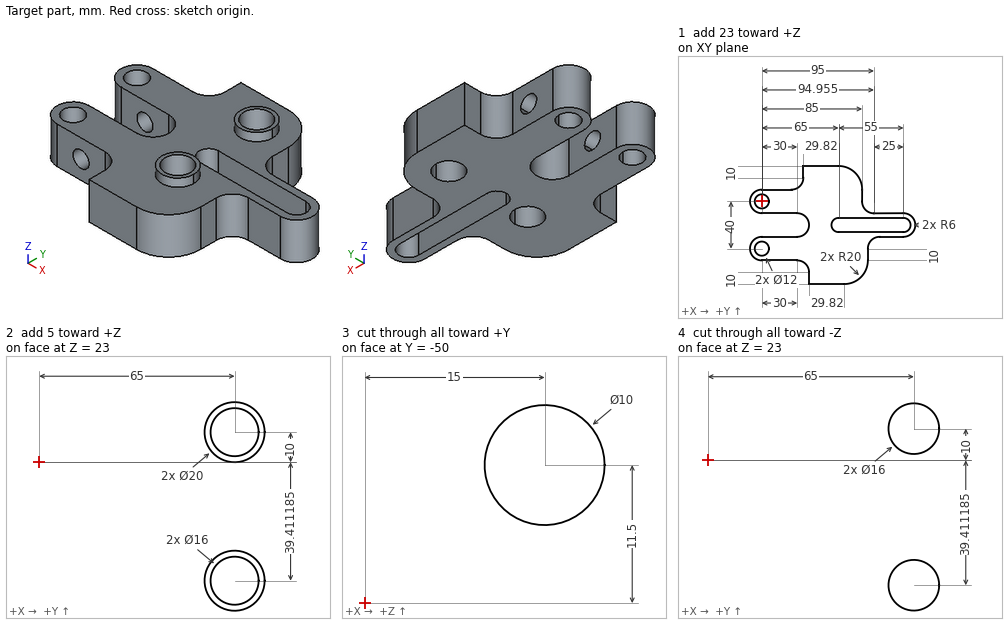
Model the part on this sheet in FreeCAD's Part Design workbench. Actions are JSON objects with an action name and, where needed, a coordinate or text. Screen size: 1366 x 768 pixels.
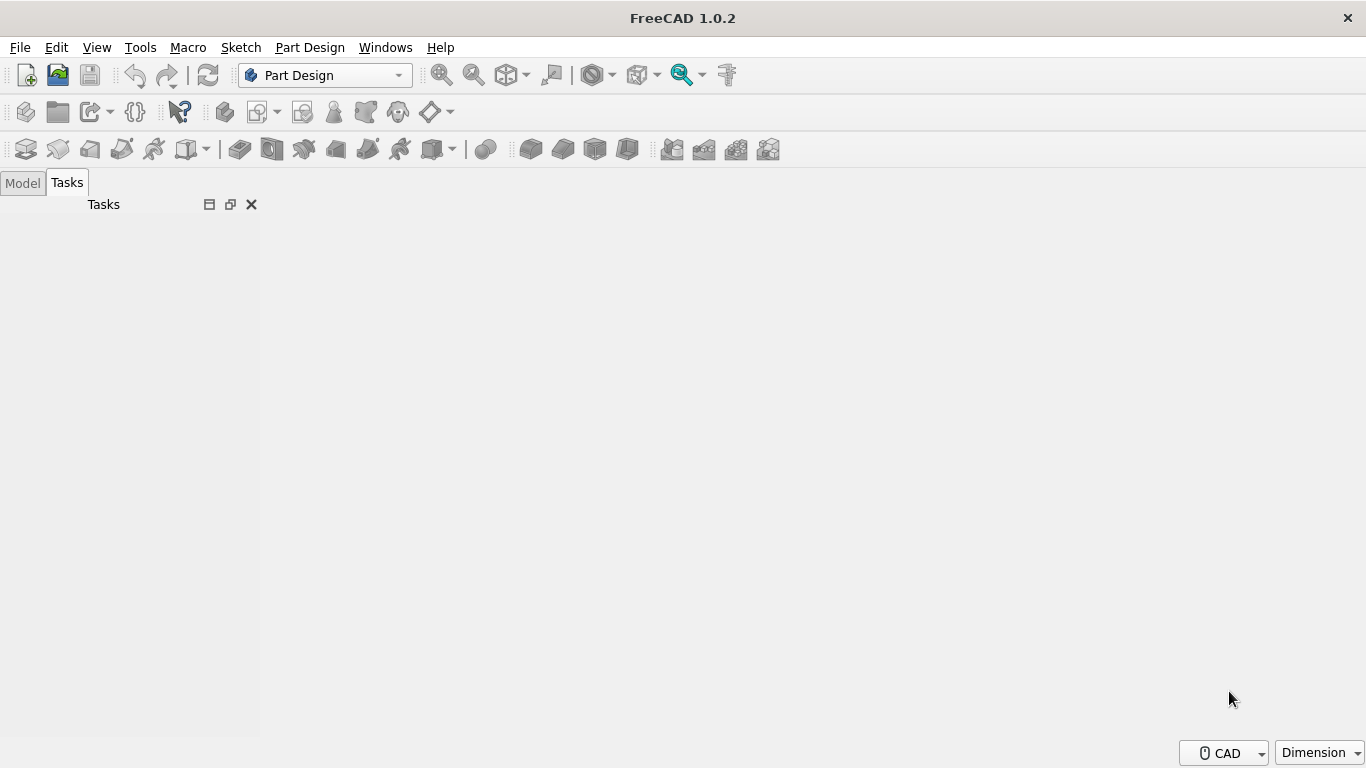
{"action": "left_click", "coordinate": [26, 76]}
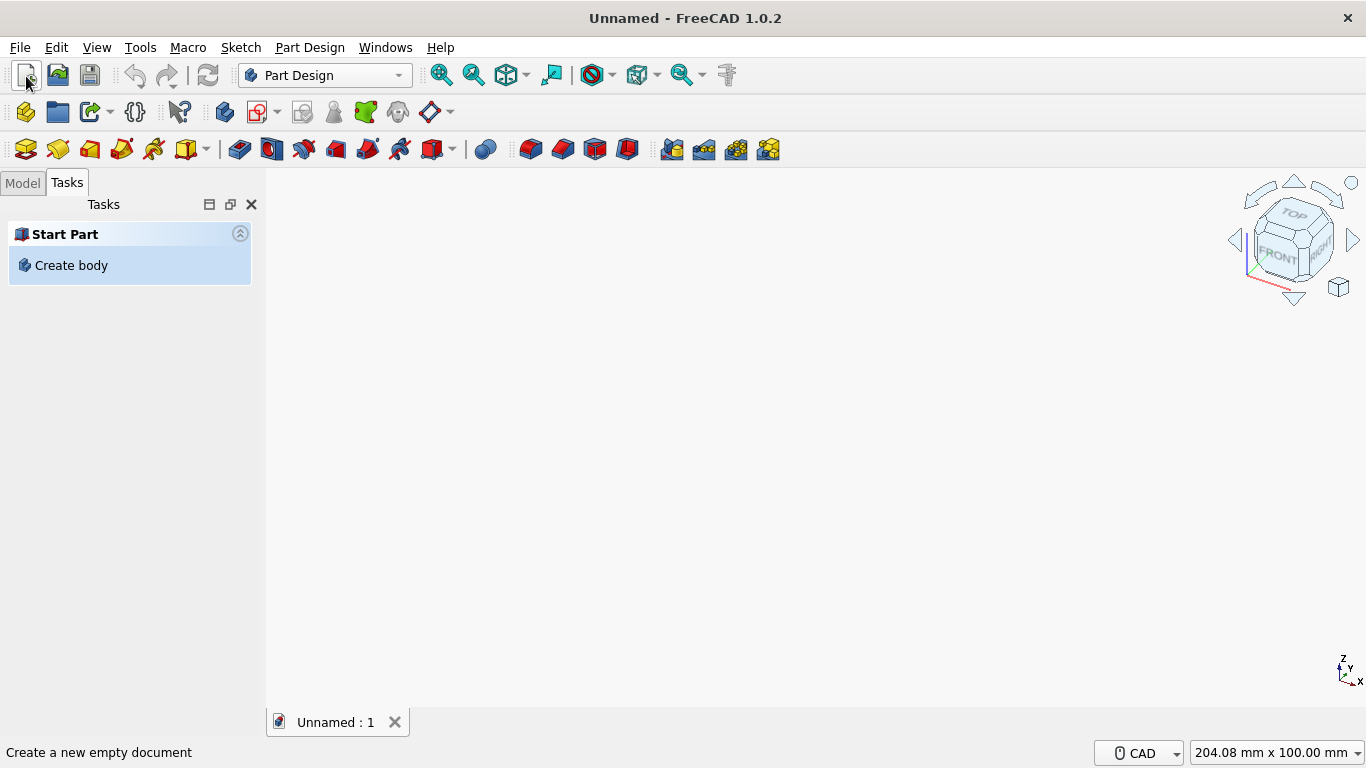
{"action": "left_click", "coordinate": [258, 112]}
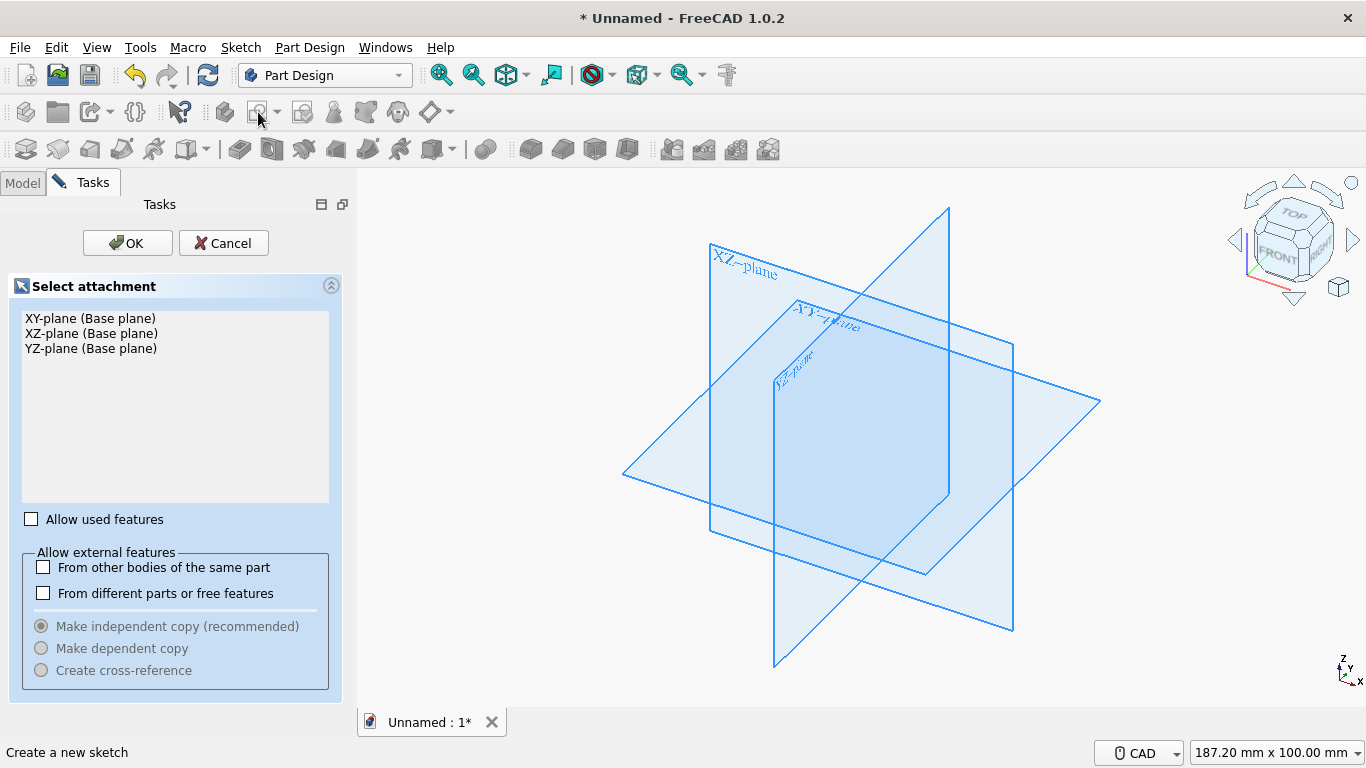
{"action": "left_click", "coordinate": [82, 318]}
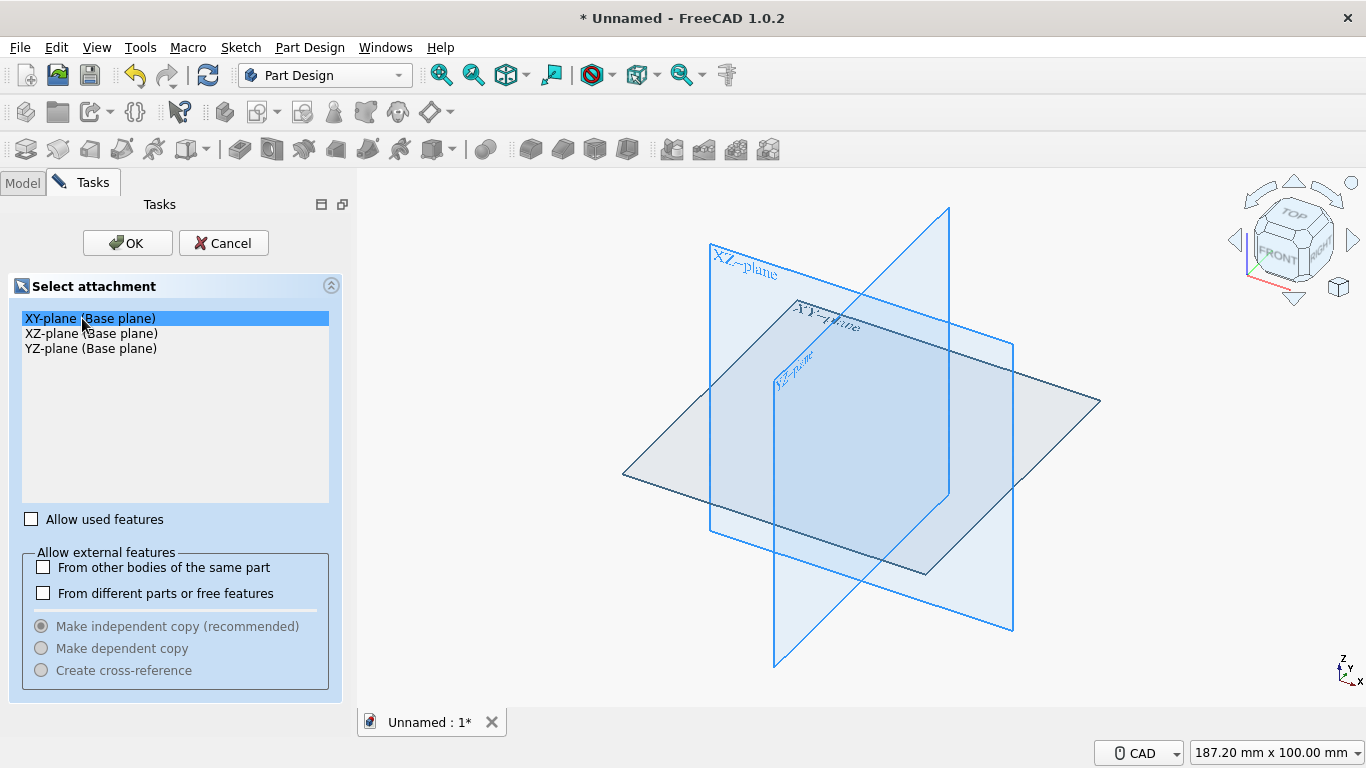
{"action": "left_click", "coordinate": [128, 243]}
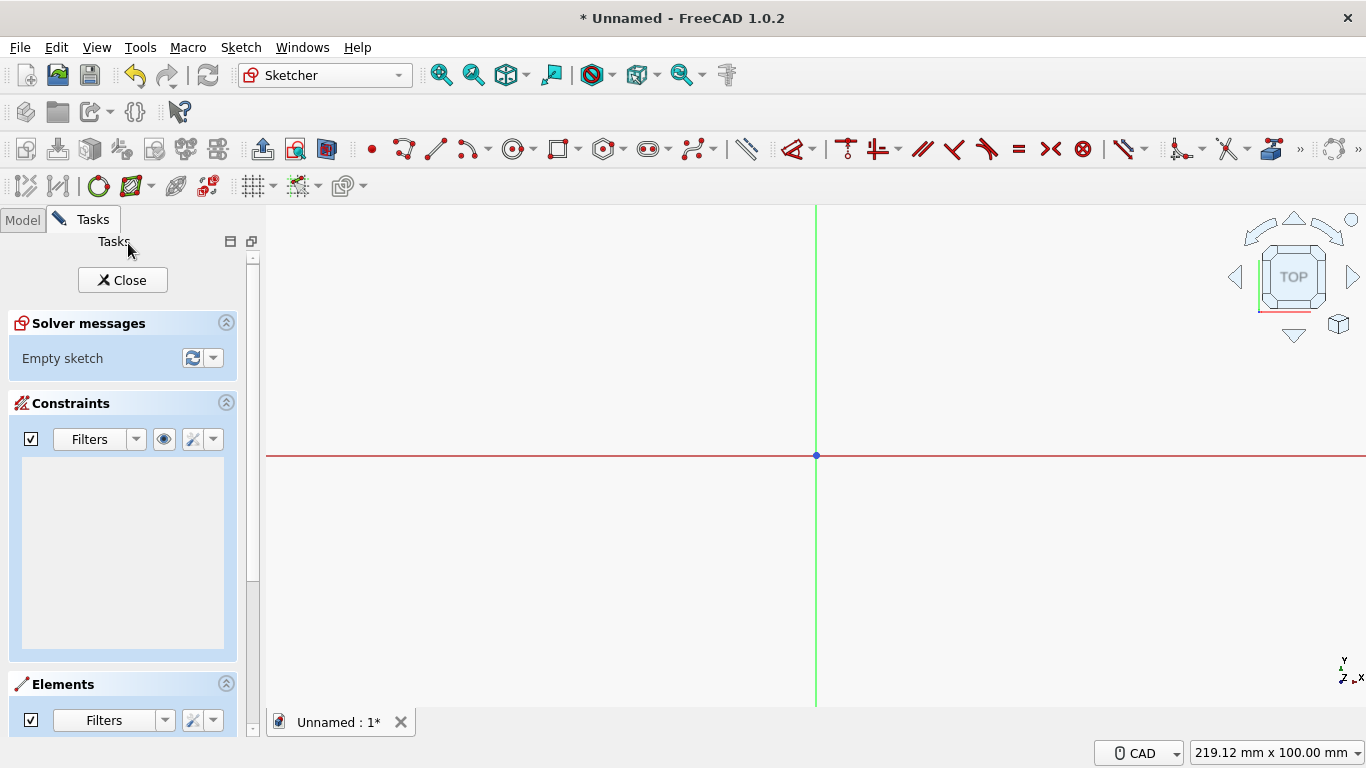
{"action": "scroll", "coordinate": [294, 252], "scroll_direction": "down", "scroll_amount": 2}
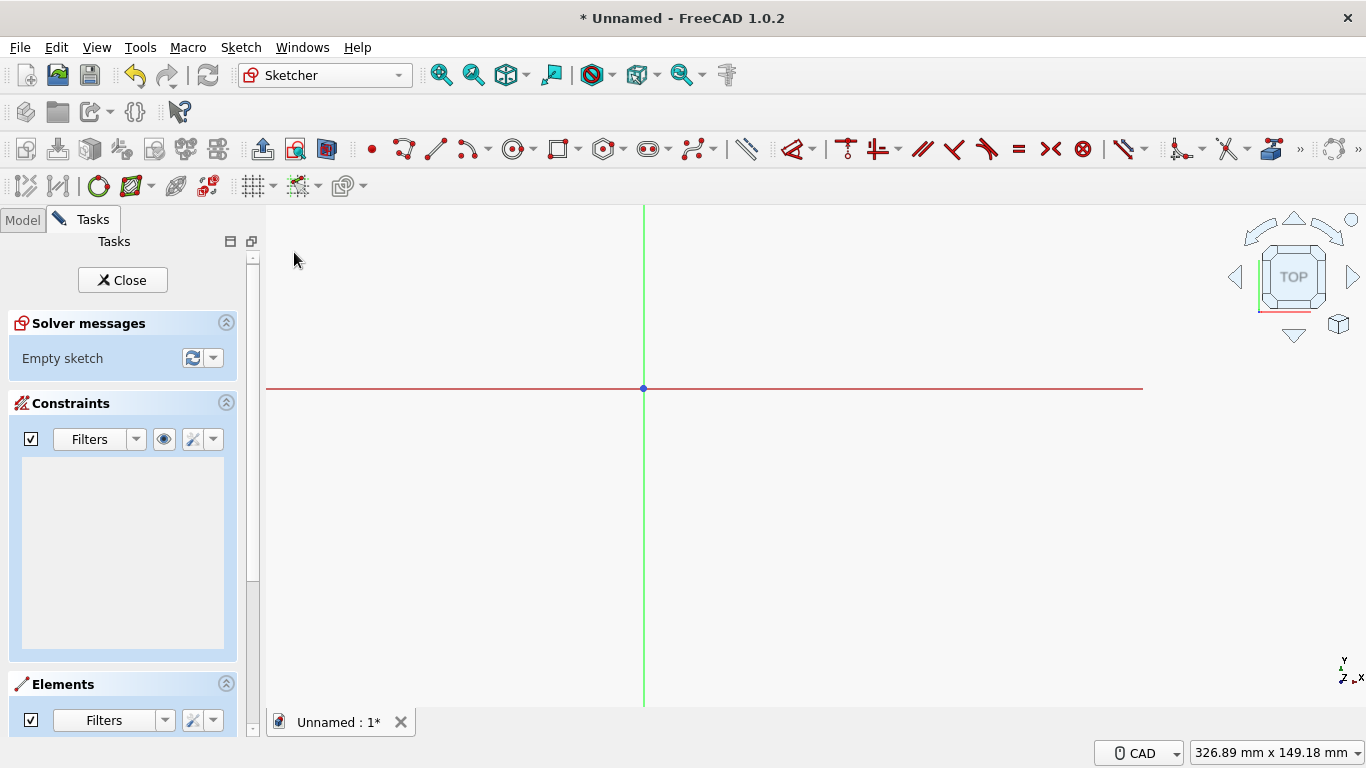
{"action": "left_click", "coordinate": [404, 150]}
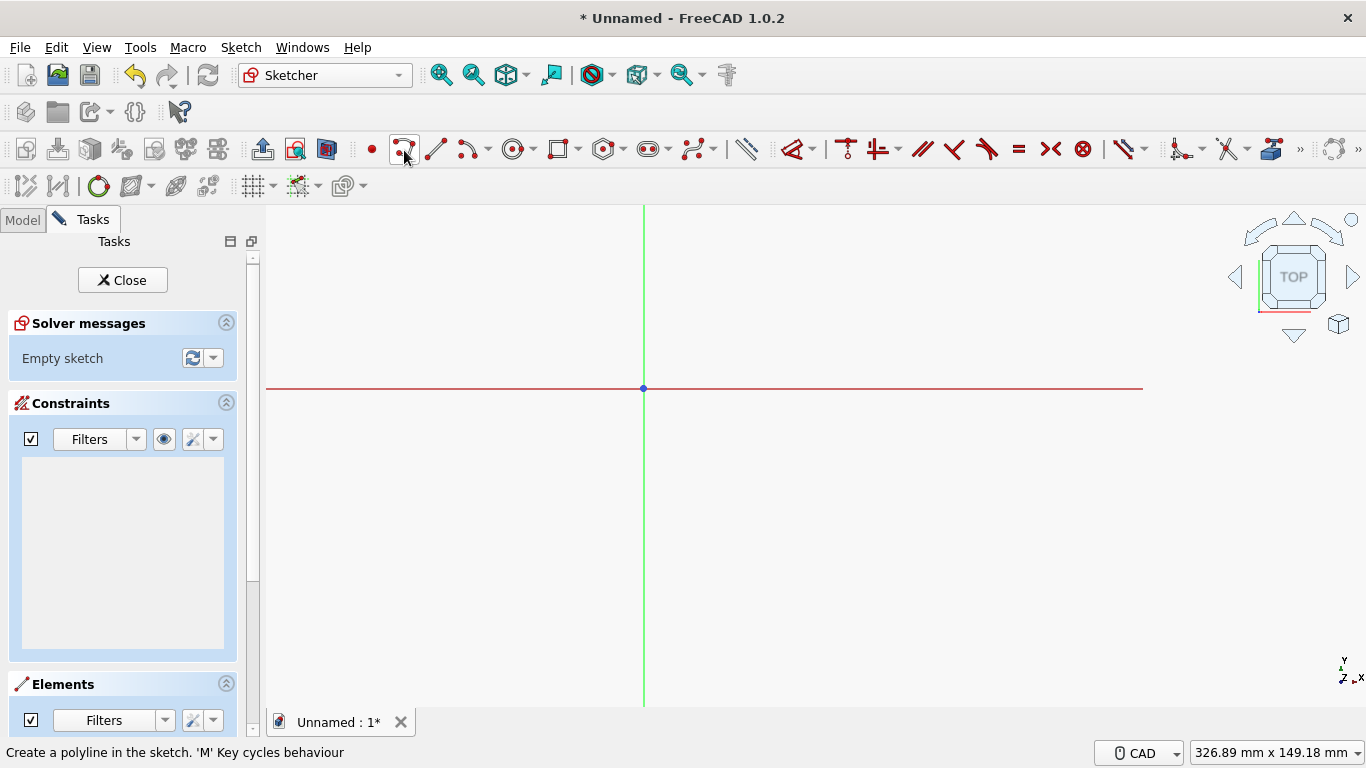
{"action": "left_click", "coordinate": [779, 591]}
{"action": "left_click", "coordinate": [779, 624]}
{"action": "left_click", "coordinate": [879, 624]}
{"action": "right_click", "coordinate": [879, 624]}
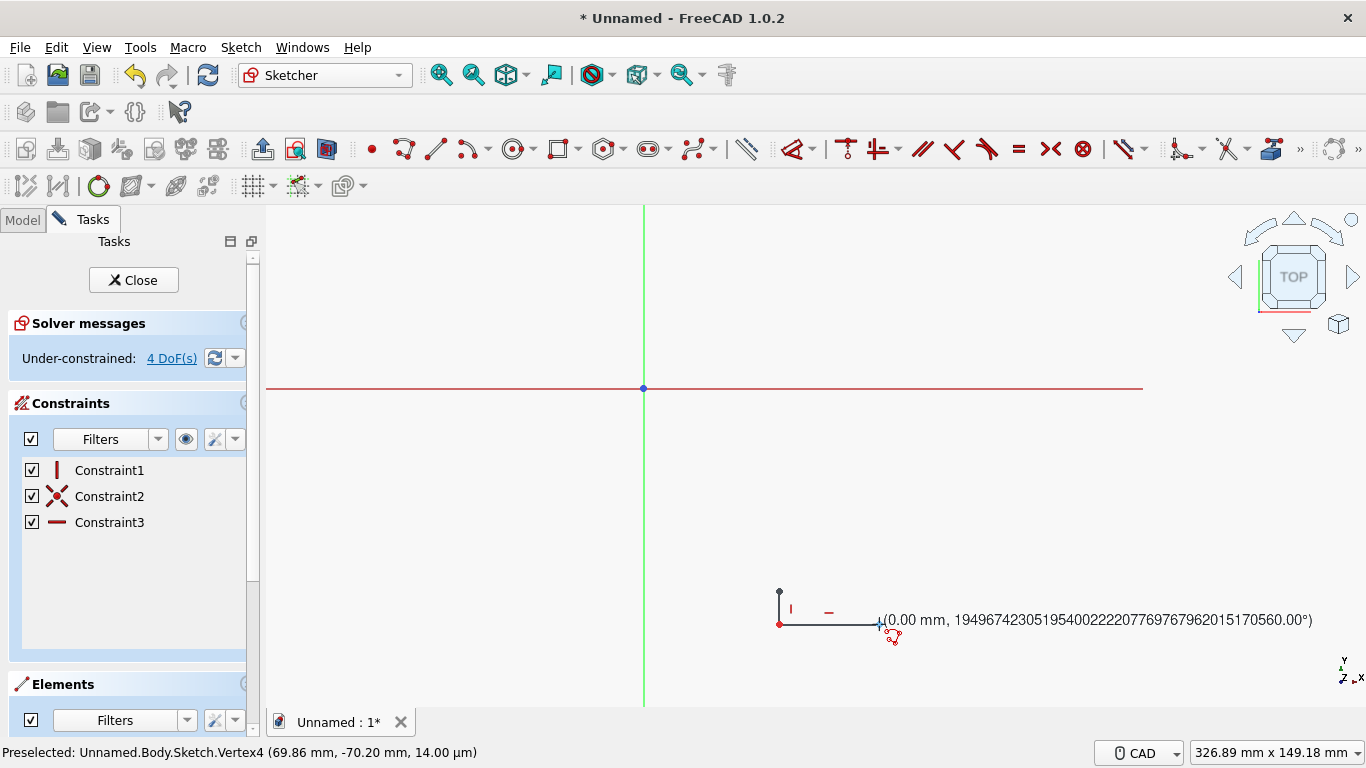
{"action": "key", "text": "g l"}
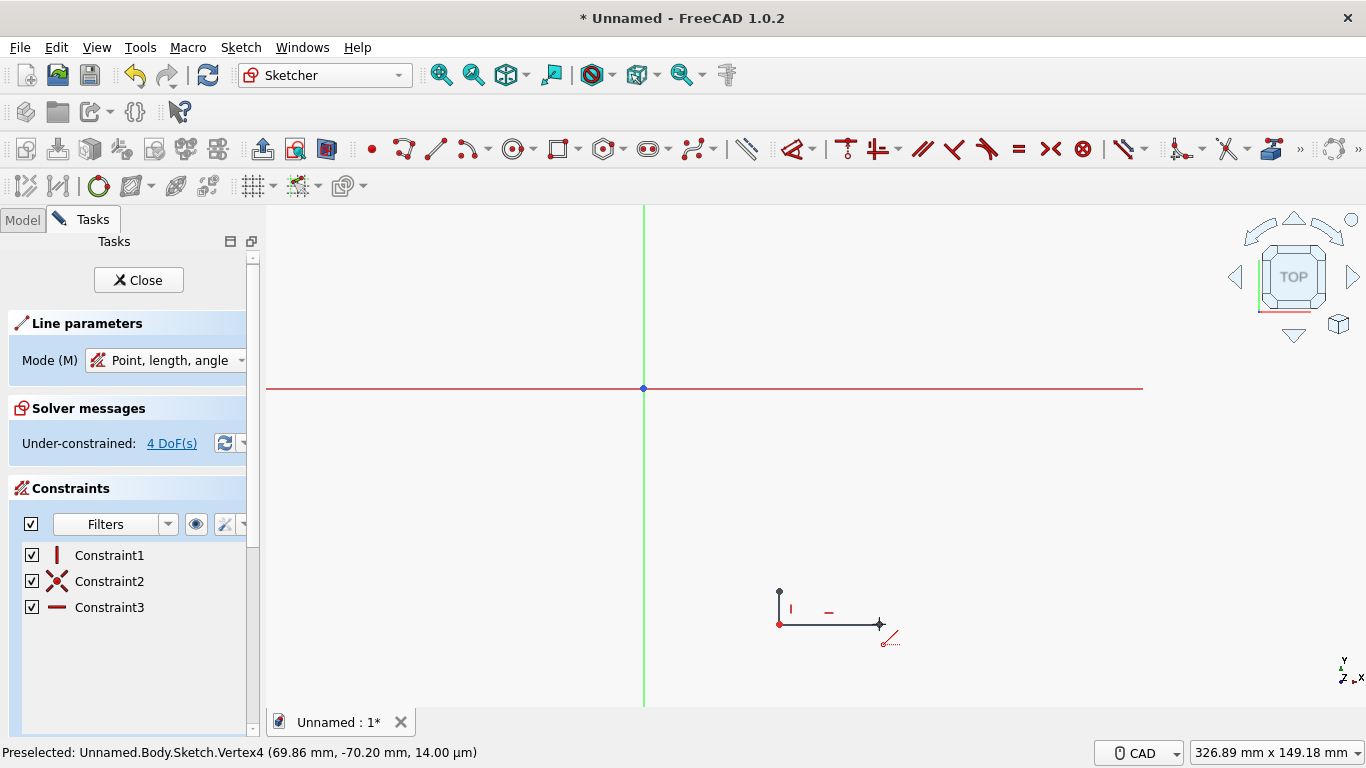
{"action": "left_click", "coordinate": [946, 557]}
{"action": "left_click", "coordinate": [946, 523]}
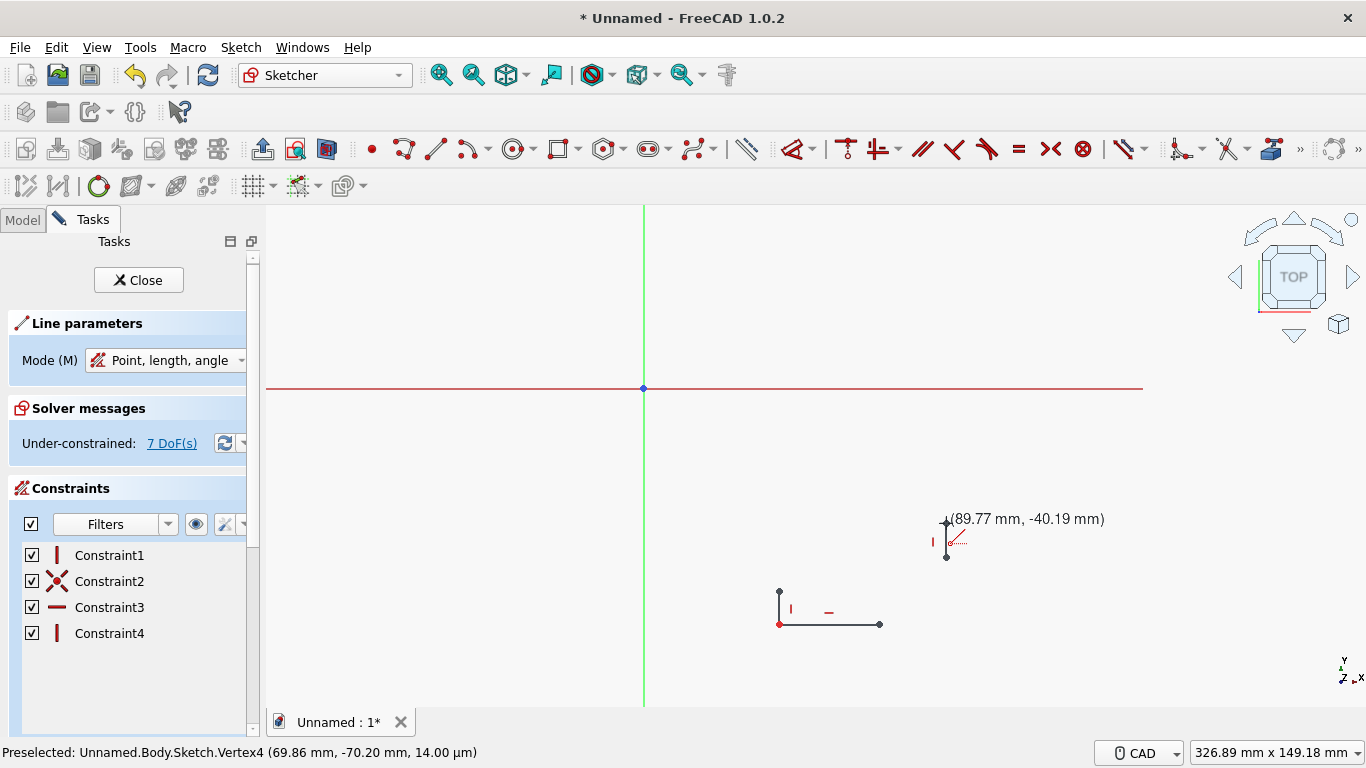
{"action": "left_click", "coordinate": [980, 490]}
{"action": "left_click", "coordinate": [1048, 490]}